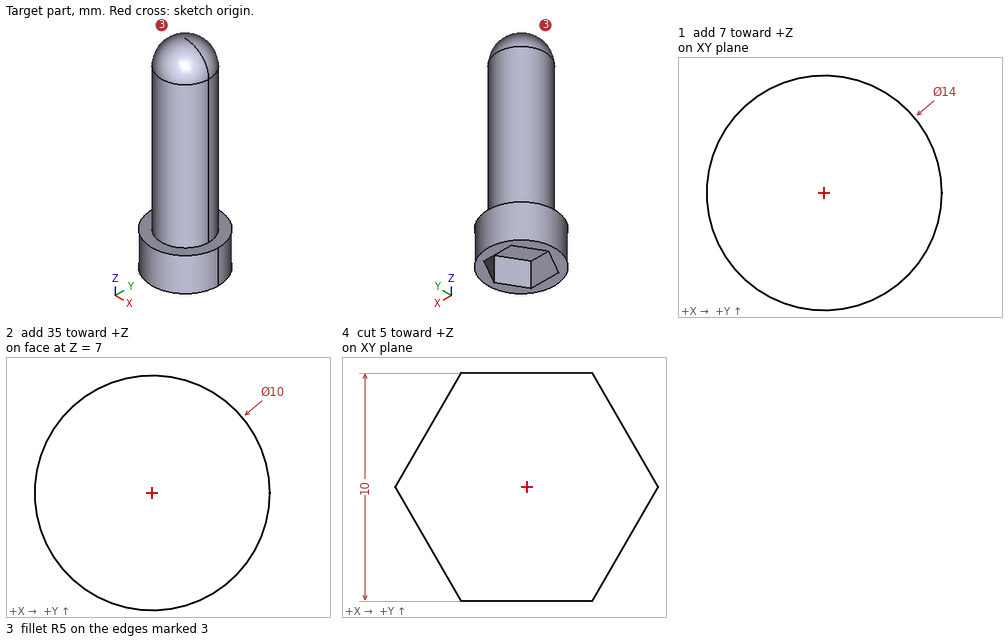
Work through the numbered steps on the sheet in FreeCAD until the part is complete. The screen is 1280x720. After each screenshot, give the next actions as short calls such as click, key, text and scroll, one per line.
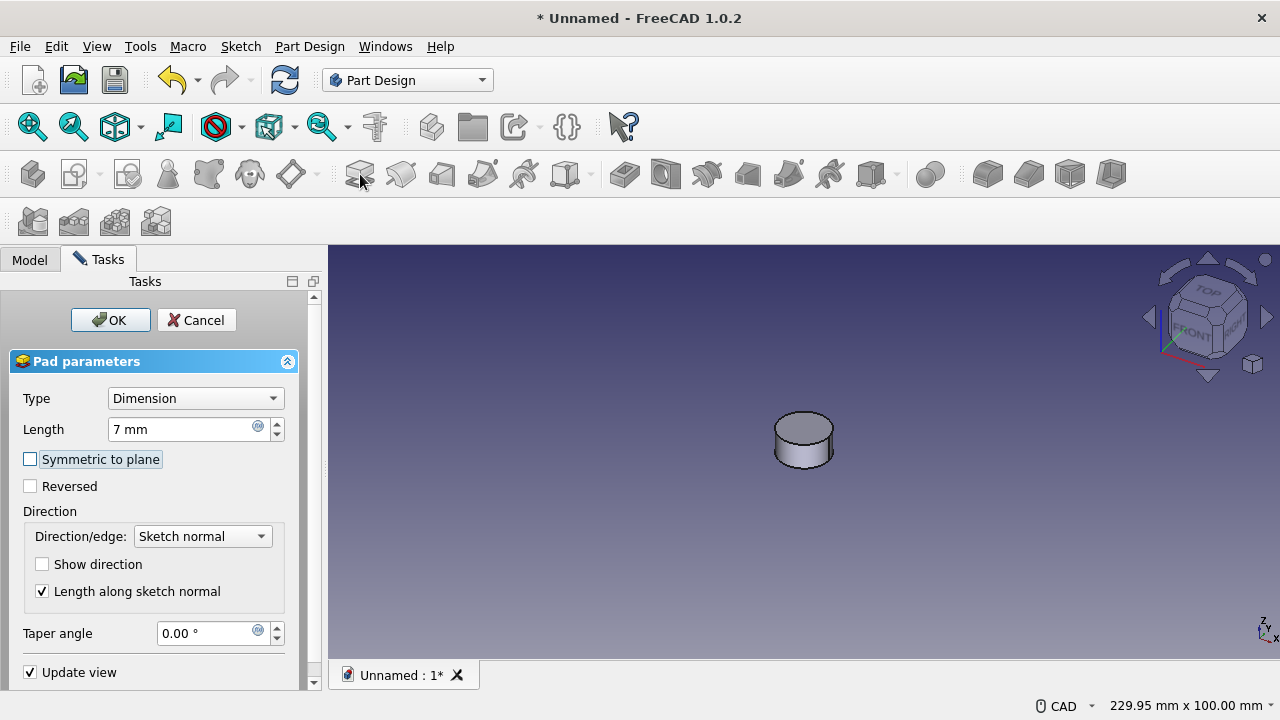
click(111, 320)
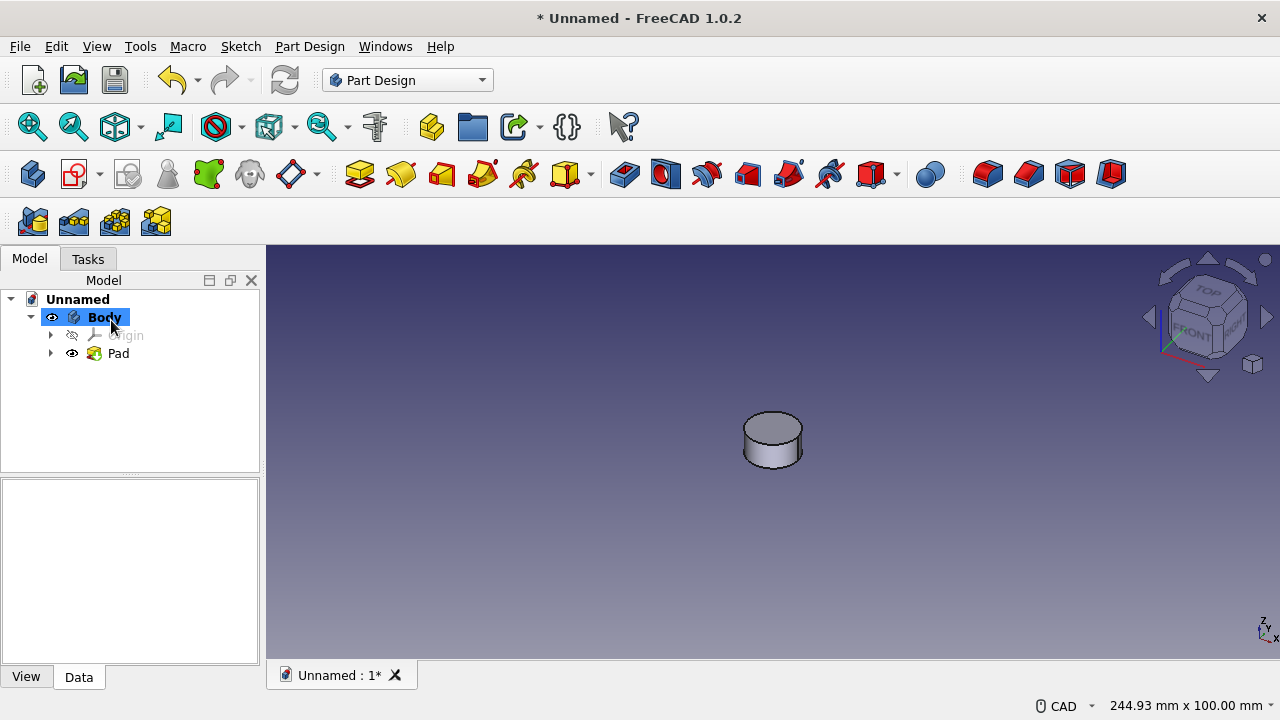
key(v)
key(f)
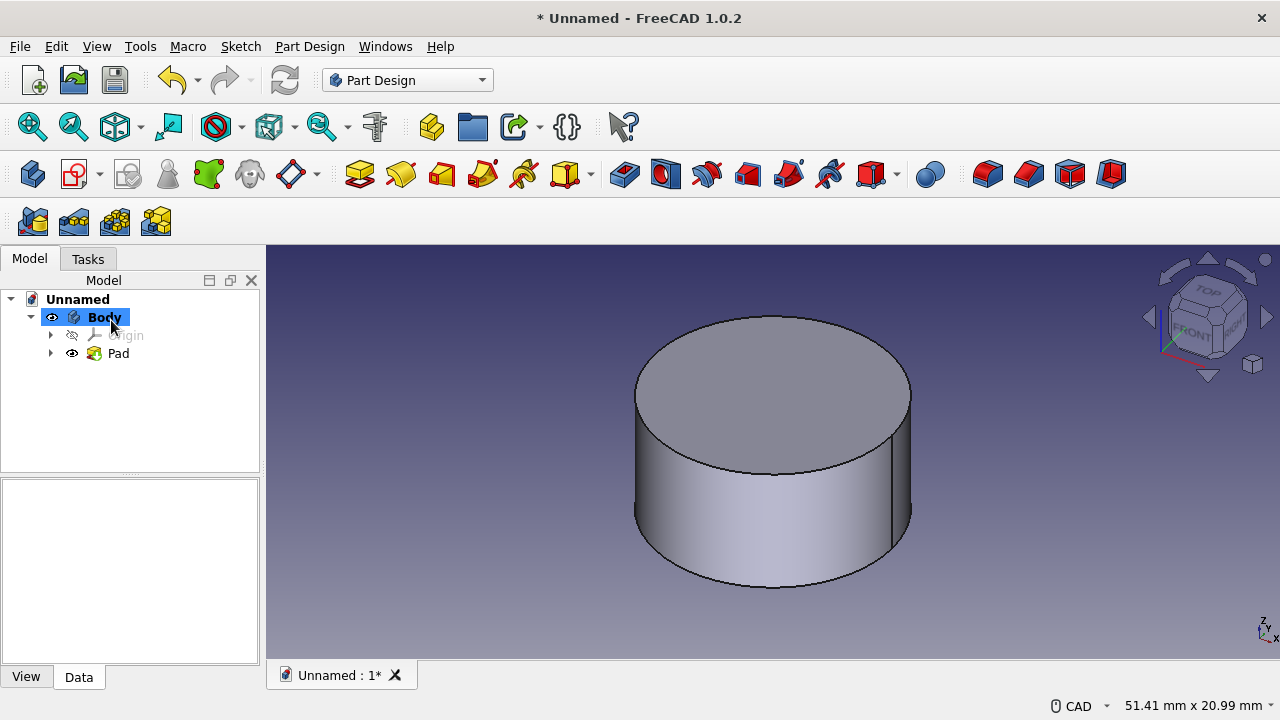
click(773, 394)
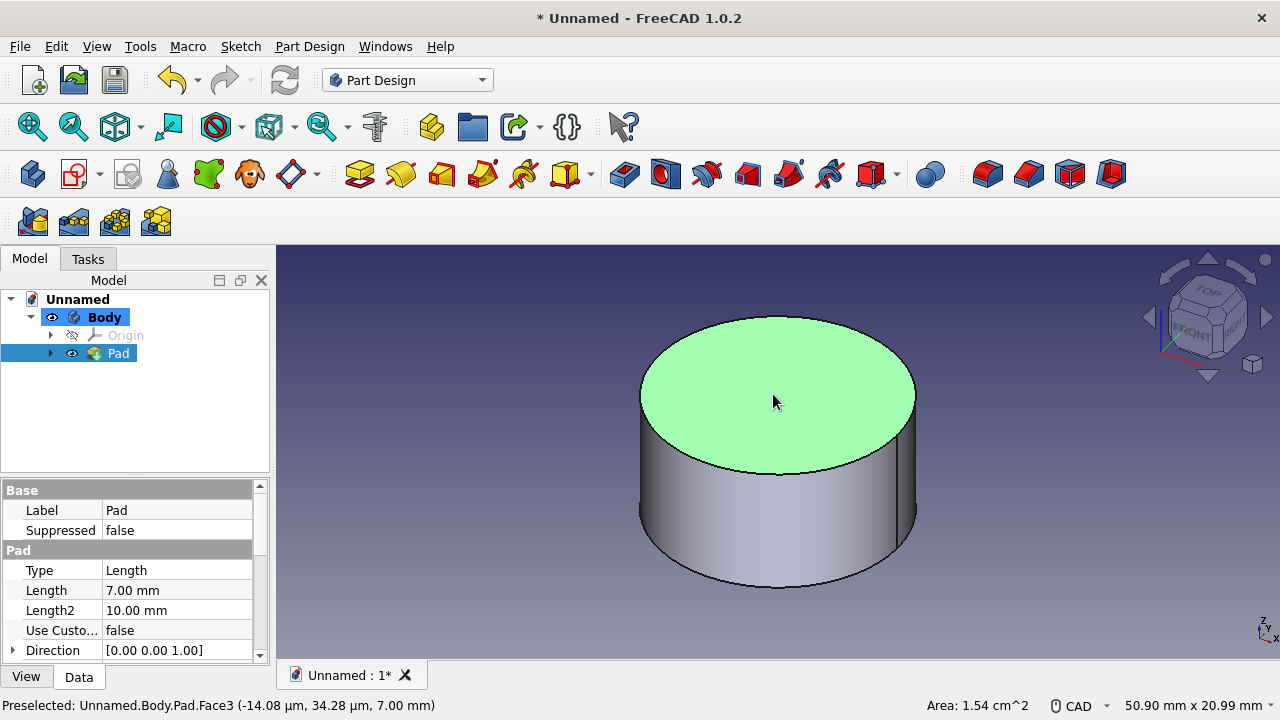
click(74, 174)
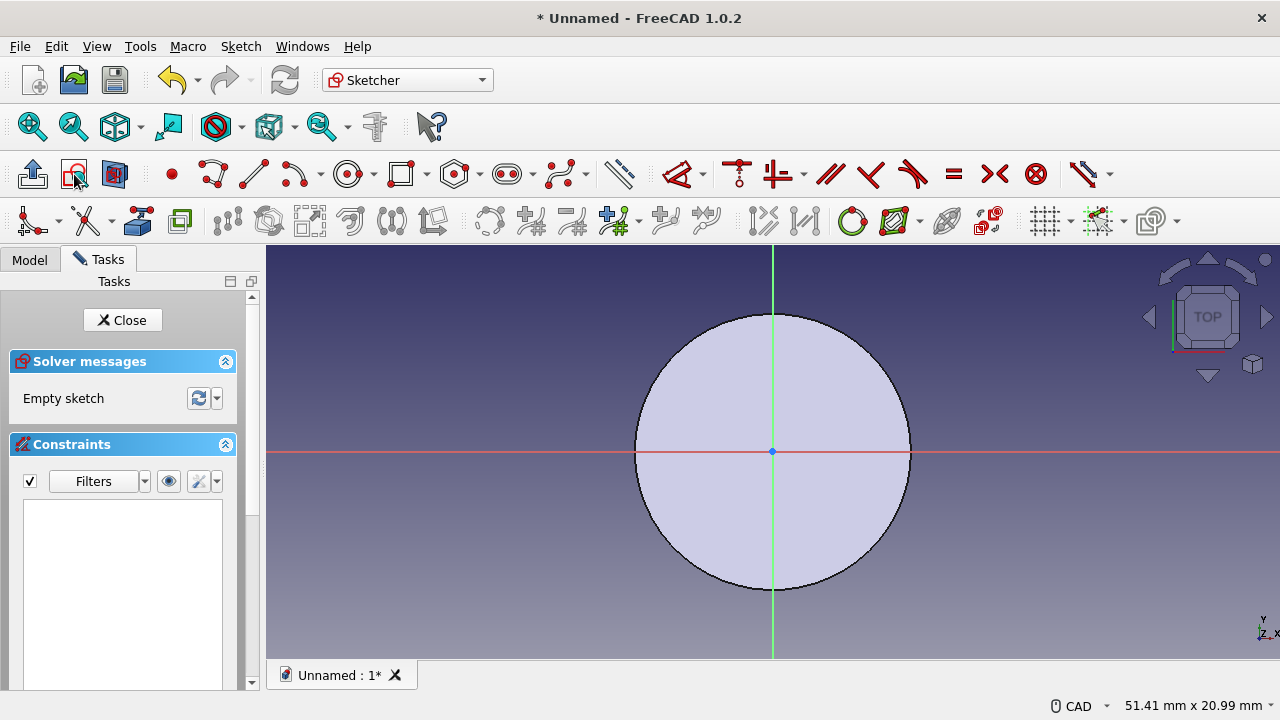
click(348, 174)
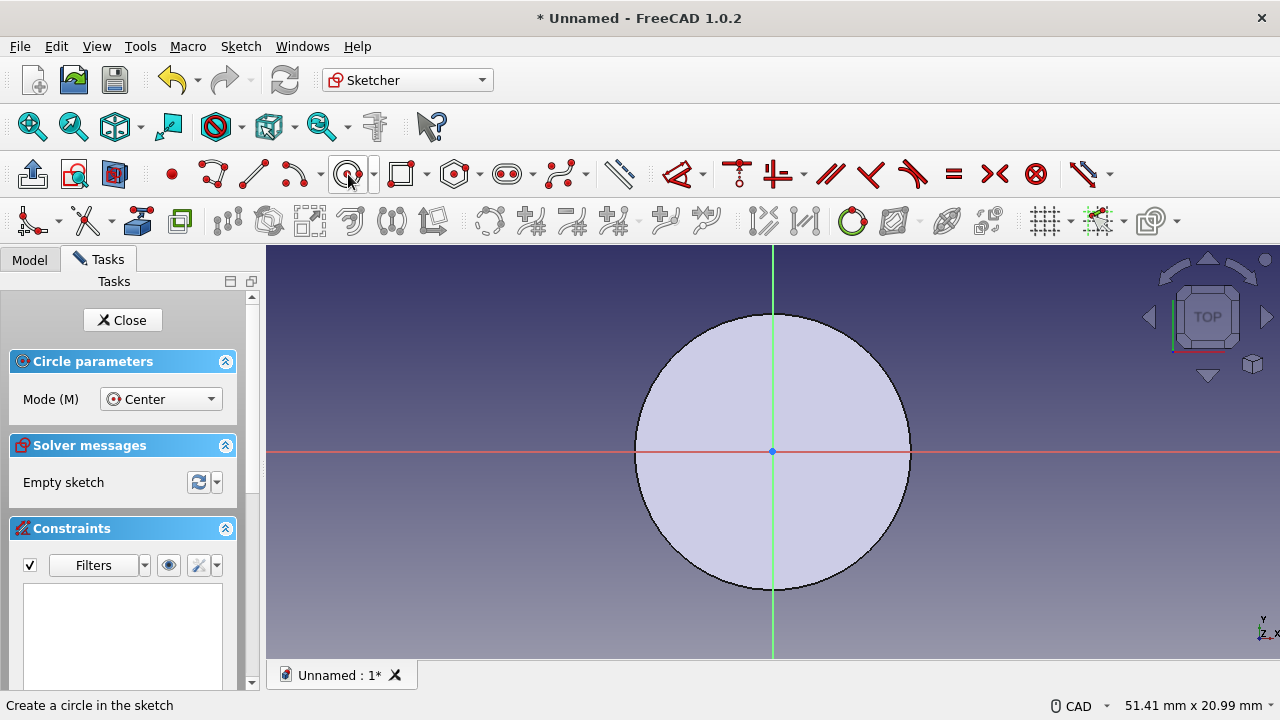
click(773, 452)
move(843, 382)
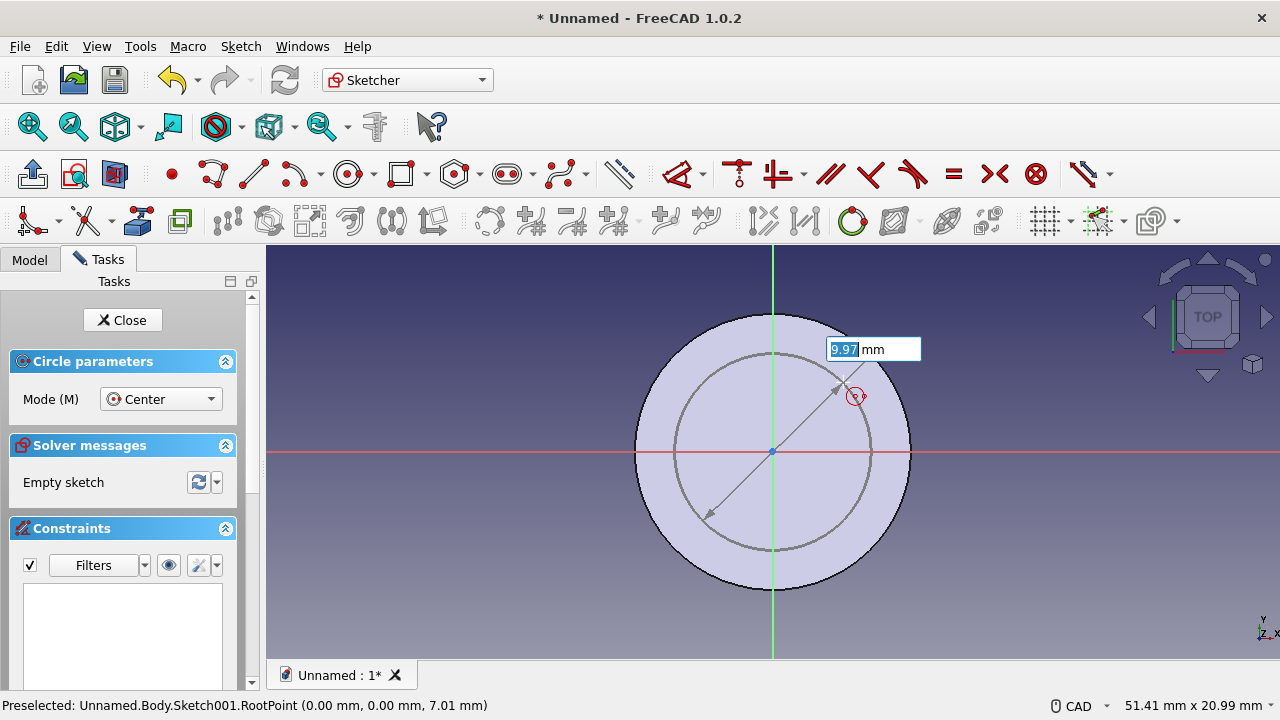
text(10)
key(Return)
key(Escape)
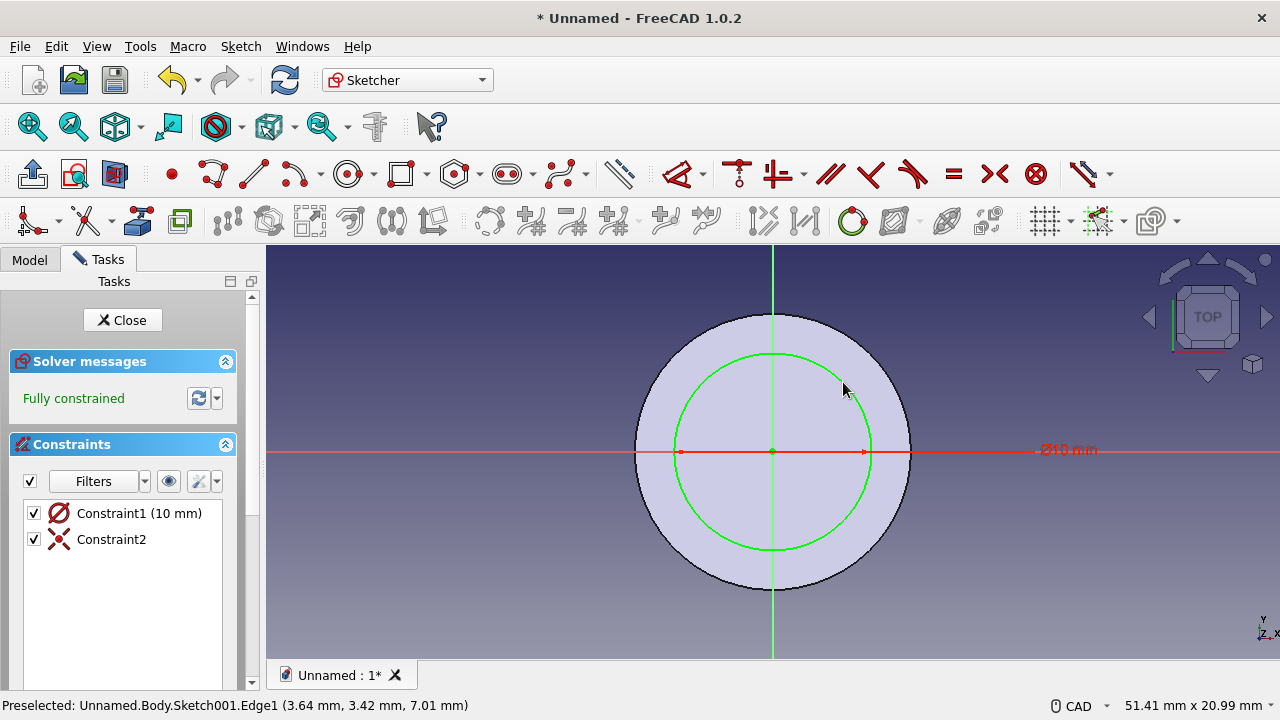
click(123, 320)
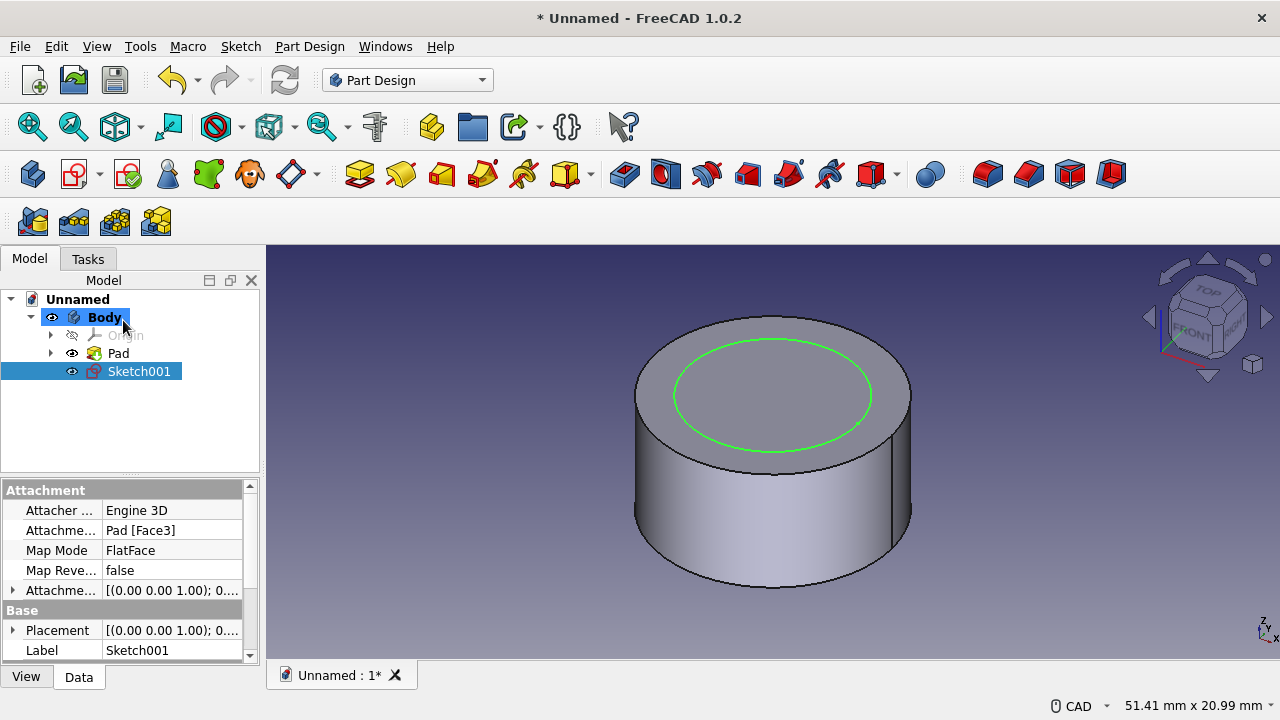
click(360, 174)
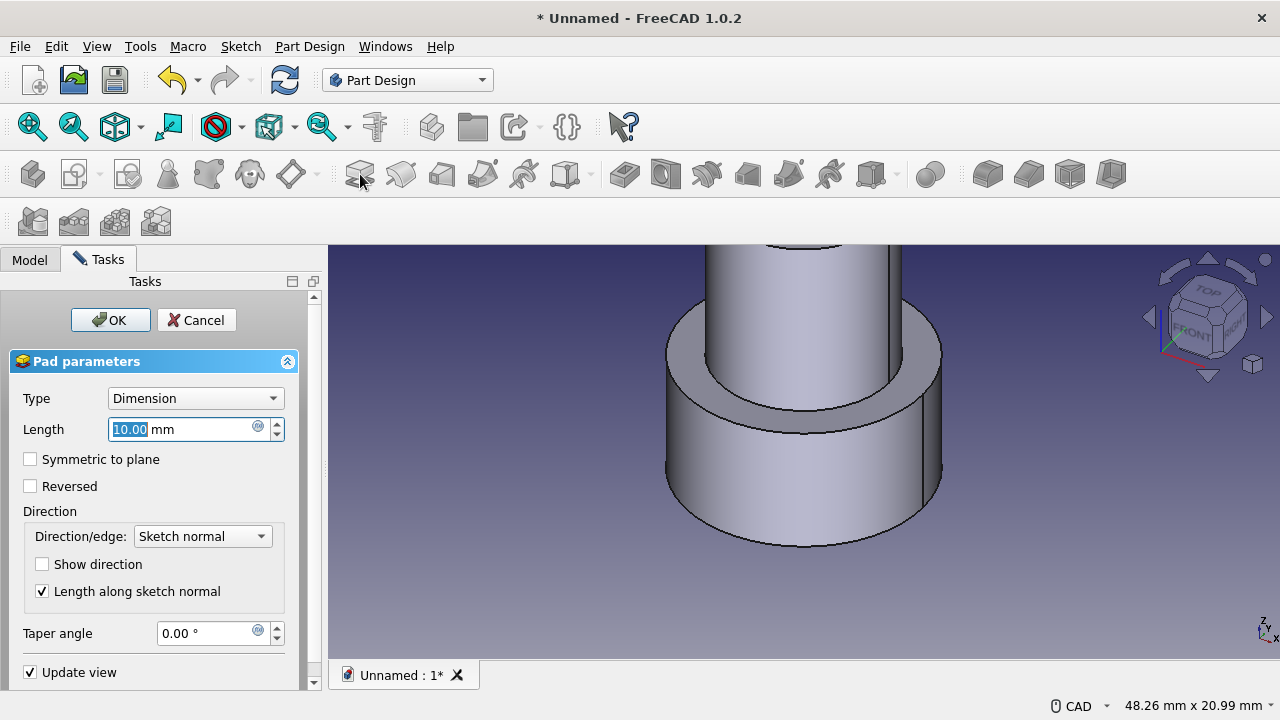
text(35)
key(Tab)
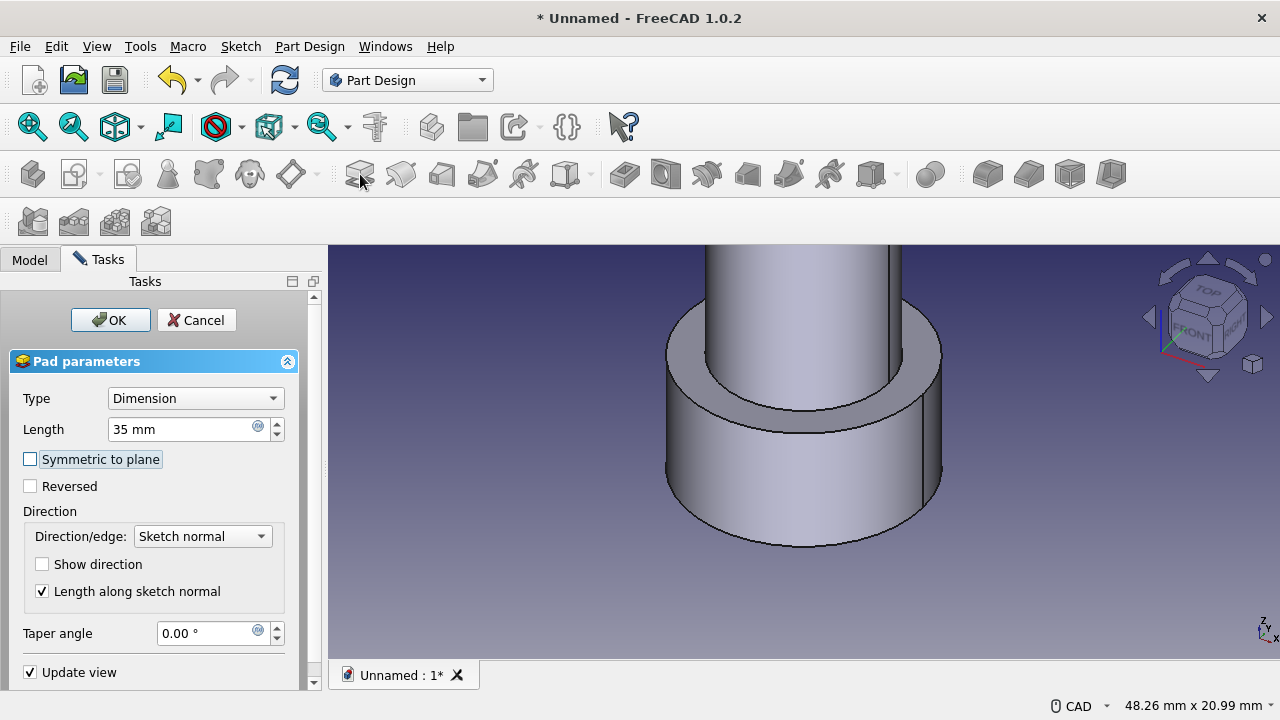
click(111, 320)